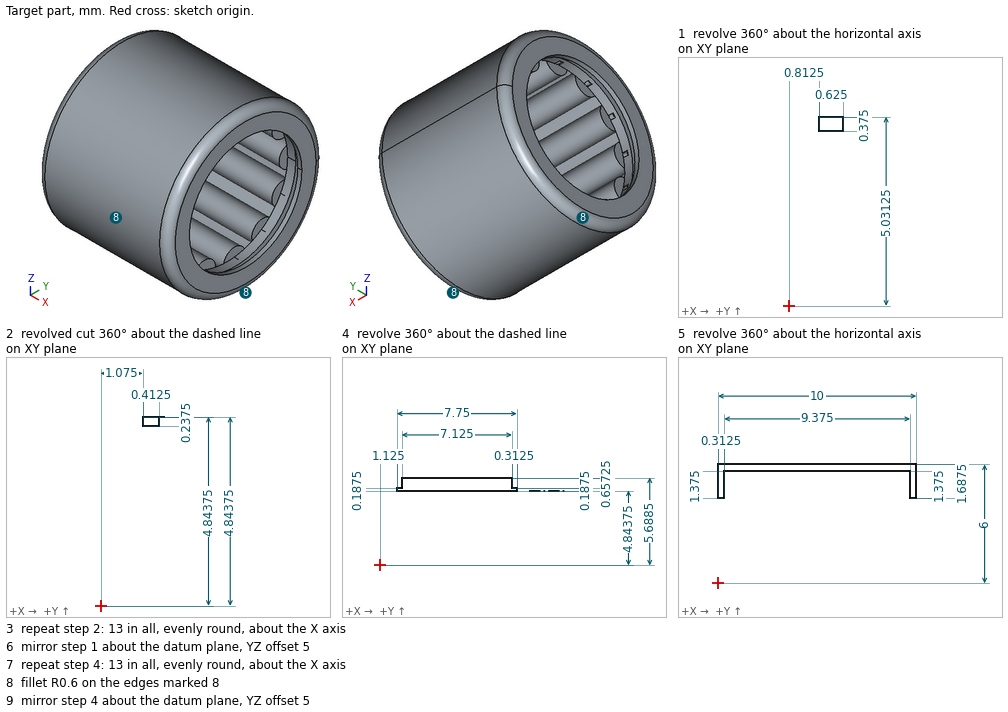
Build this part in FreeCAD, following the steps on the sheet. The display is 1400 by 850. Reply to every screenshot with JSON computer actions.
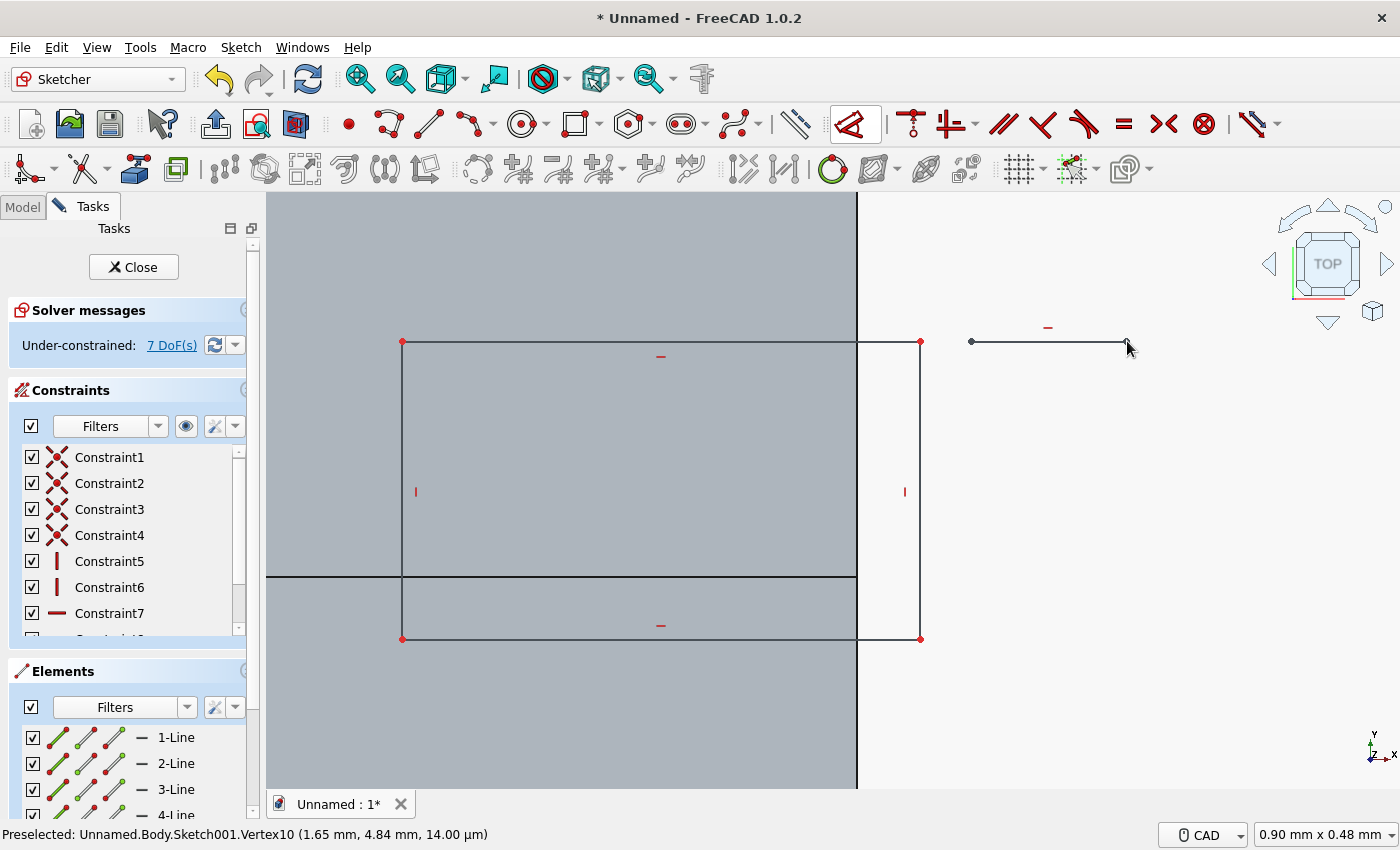
{"action": "left_click", "coordinate": [1018, 342]}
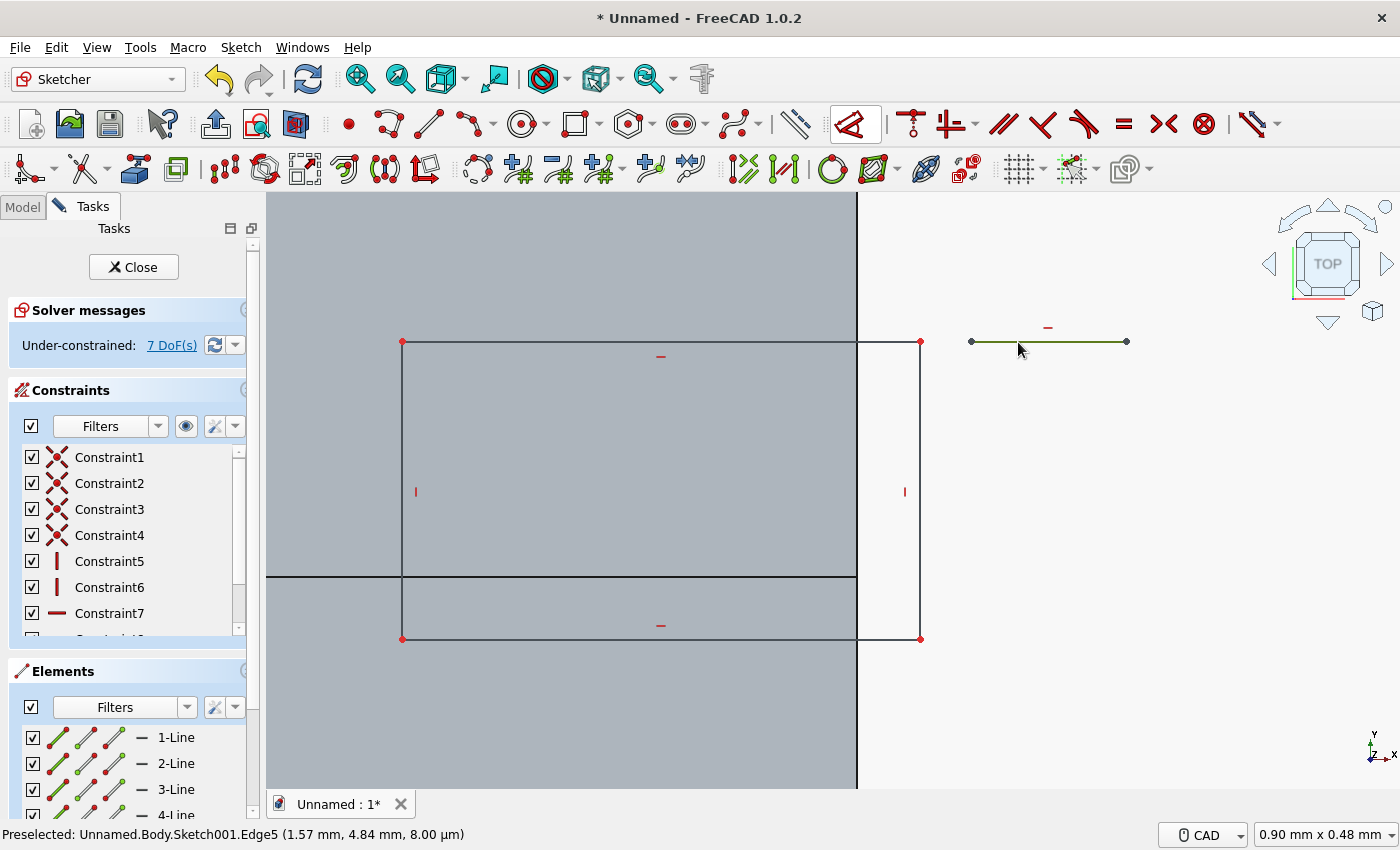
{"action": "key", "text": "g n"}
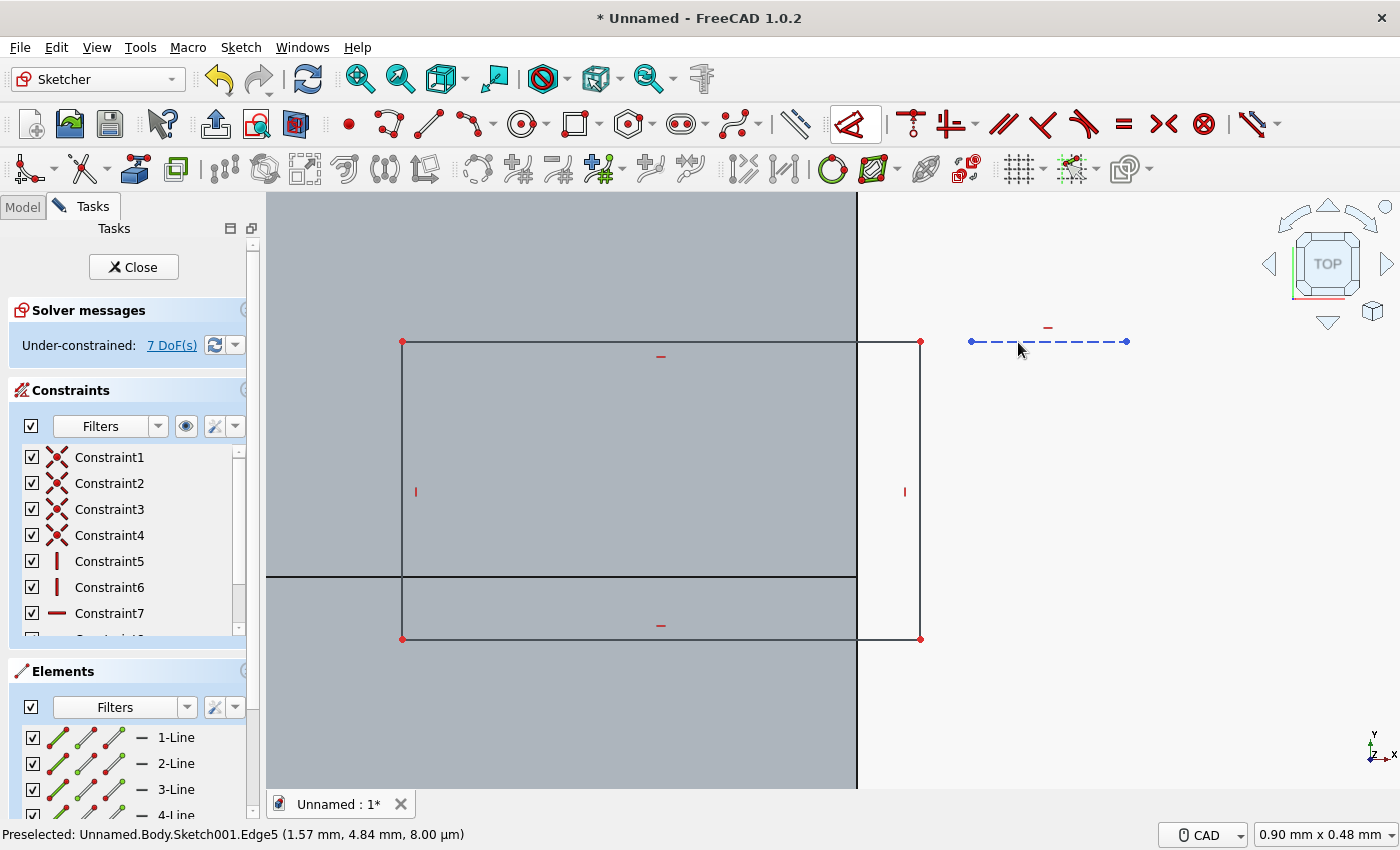
{"action": "left_click", "coordinate": [850, 124]}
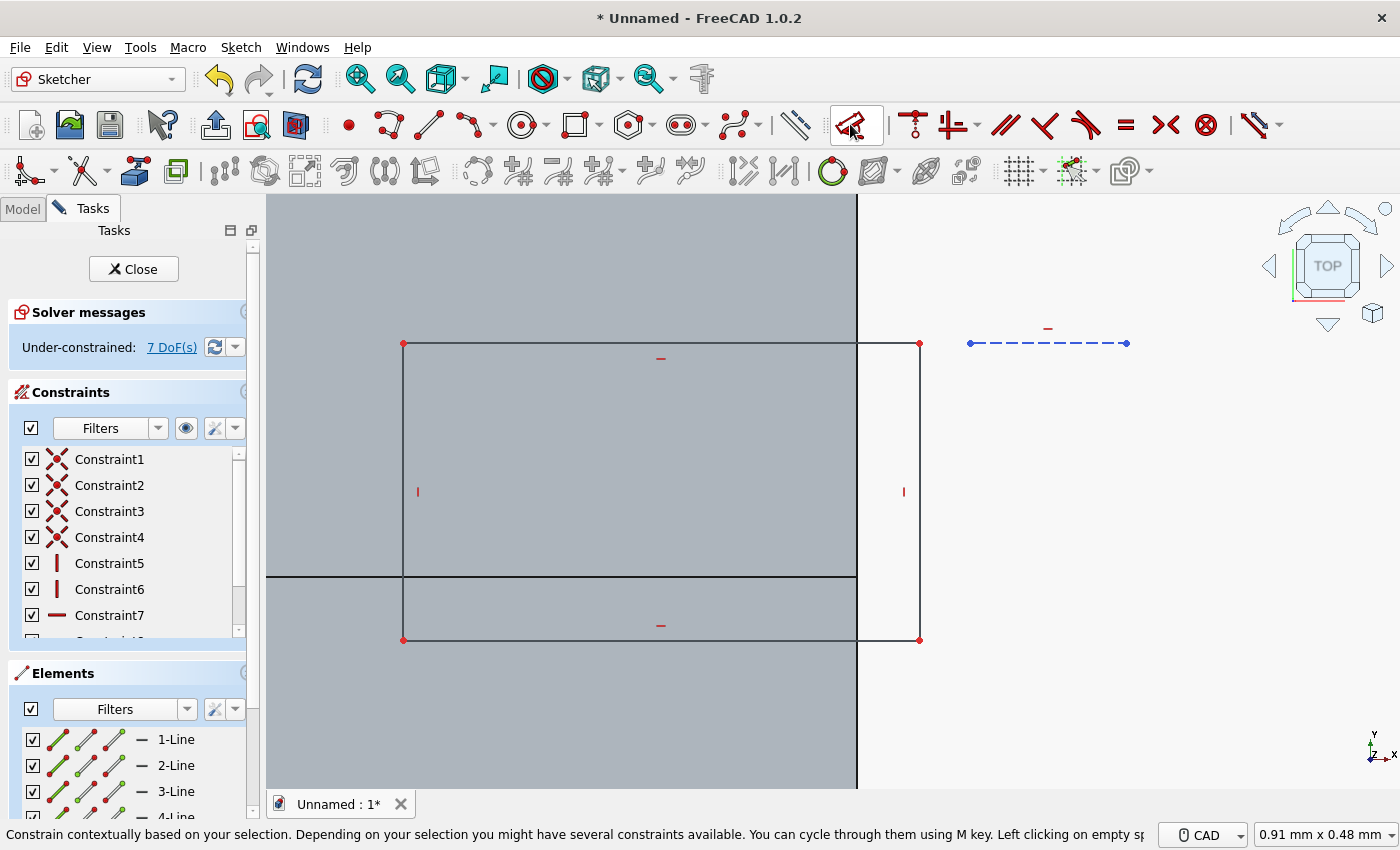
{"action": "left_click", "coordinate": [403, 433]}
{"action": "left_click", "coordinate": [369, 492]}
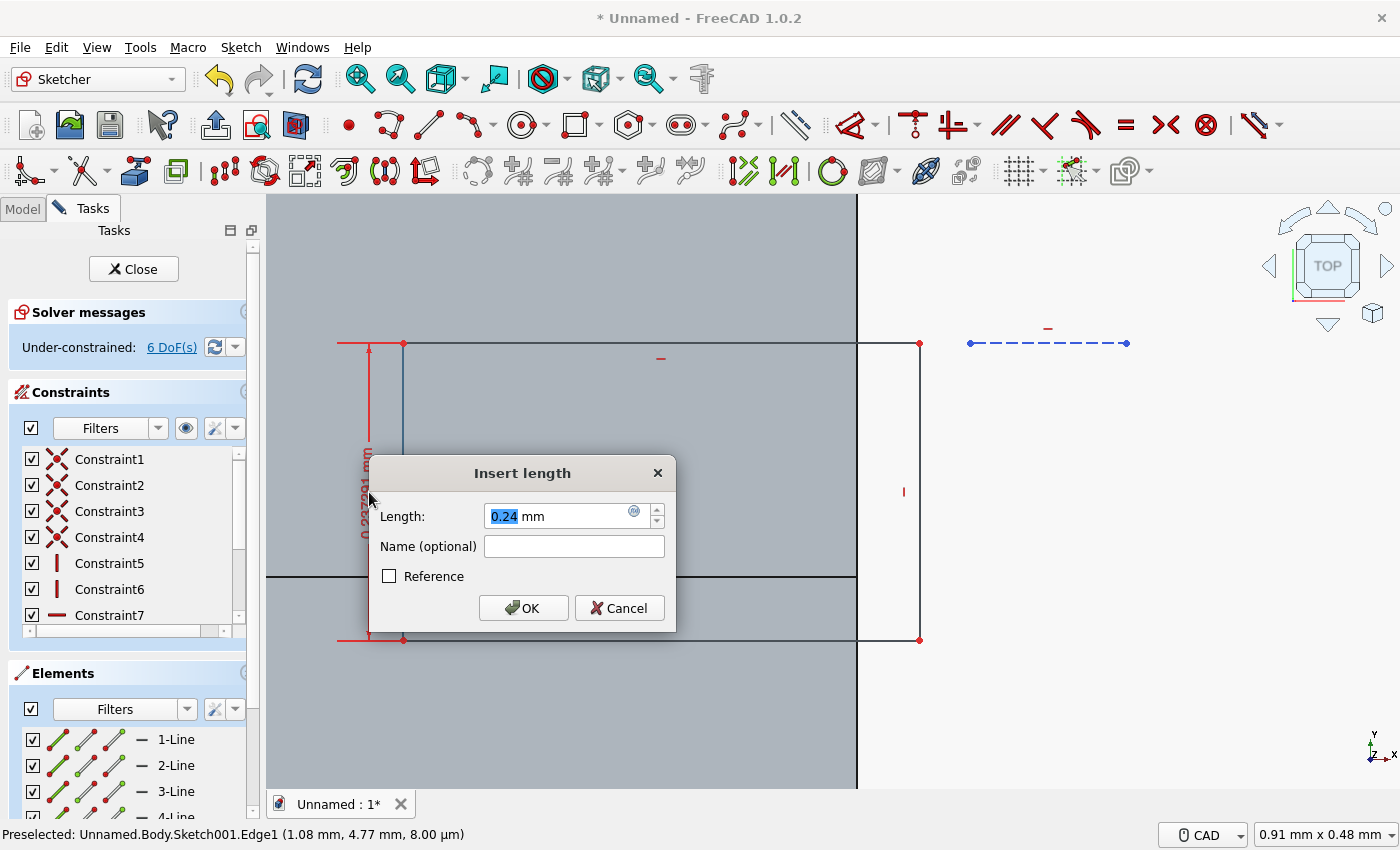
{"action": "type", "text": "0.2375"}
{"action": "key", "text": "Return"}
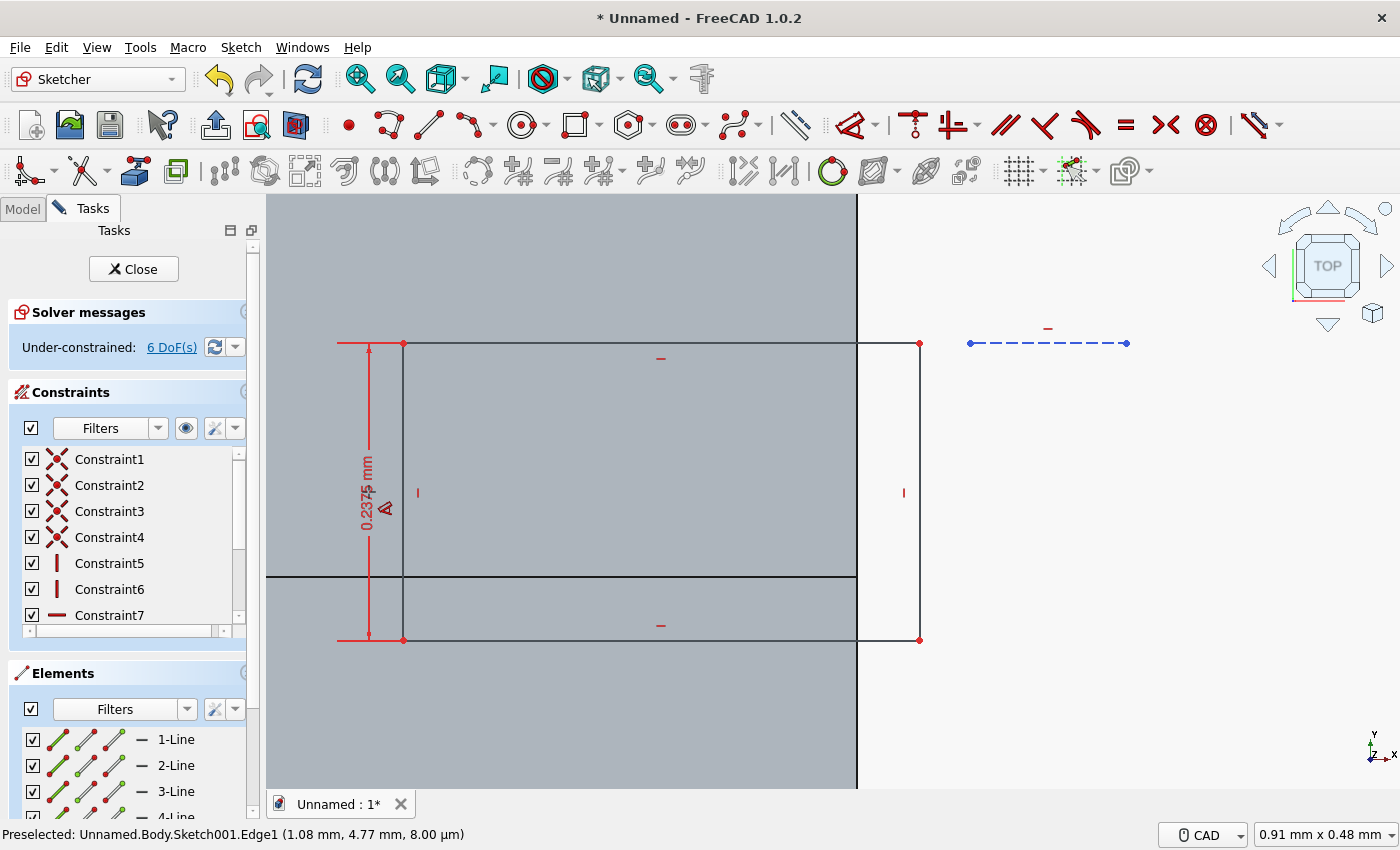
{"action": "left_click", "coordinate": [558, 641]}
{"action": "left_click", "coordinate": [662, 675]}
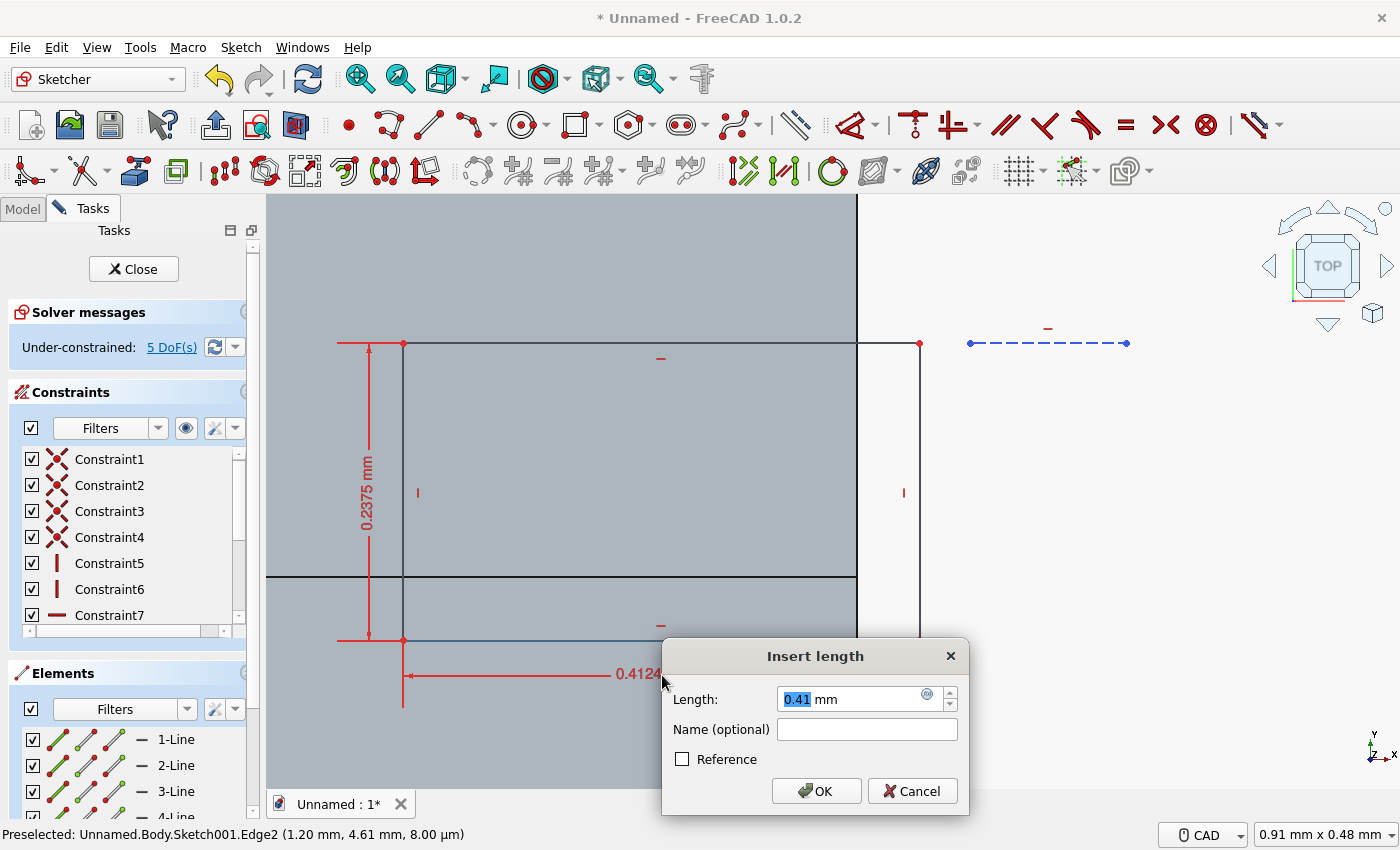
{"action": "type", "text": "0.4125"}
{"action": "key", "text": "Return"}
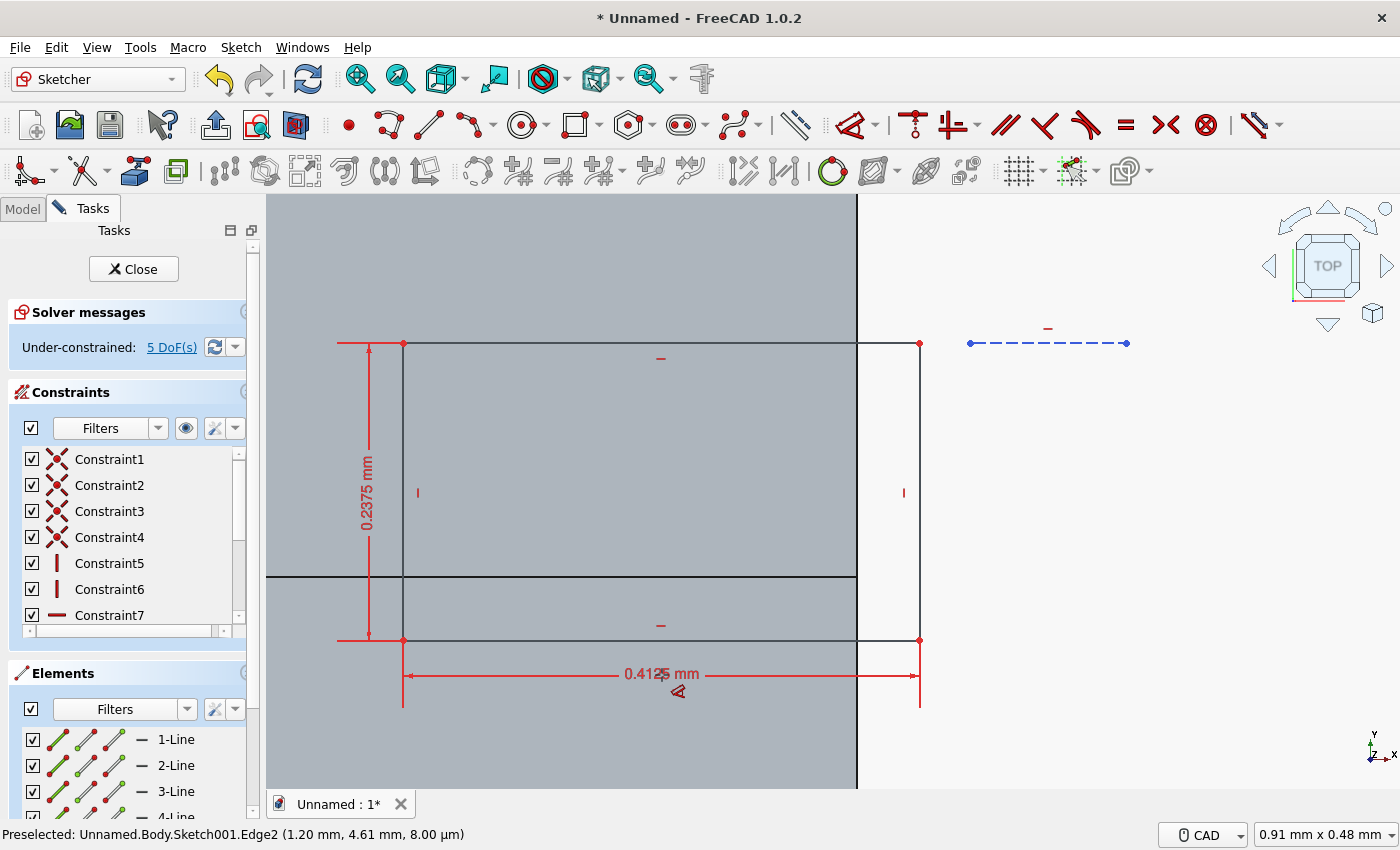
{"action": "left_click", "coordinate": [403, 343]}
{"action": "left_click", "coordinate": [349, 309]}